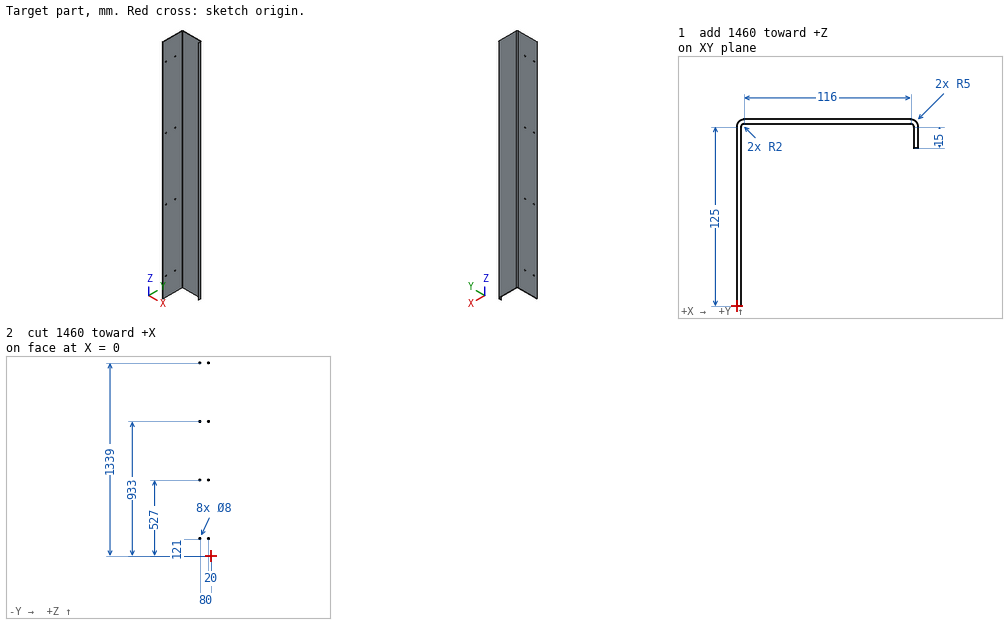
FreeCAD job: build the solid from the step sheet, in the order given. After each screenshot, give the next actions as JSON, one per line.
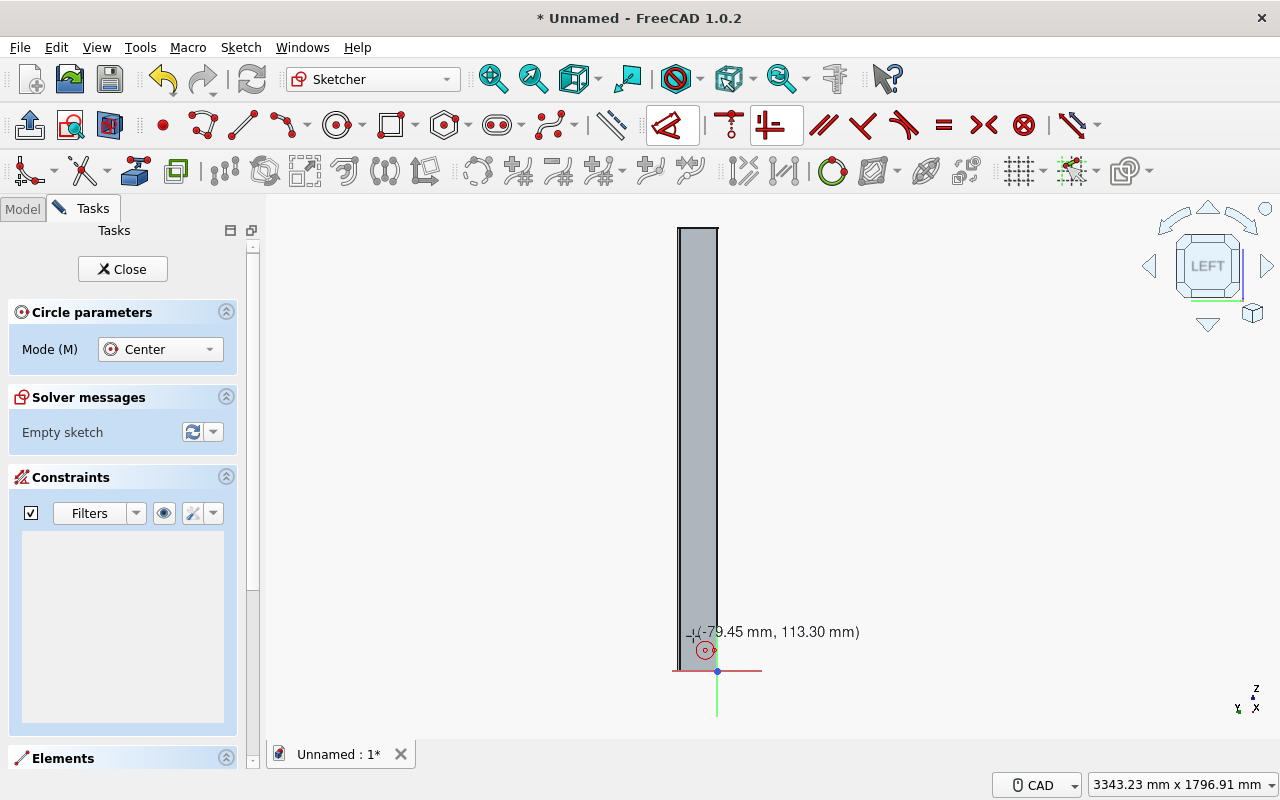
{"action": "left_click", "coordinate": [693, 634]}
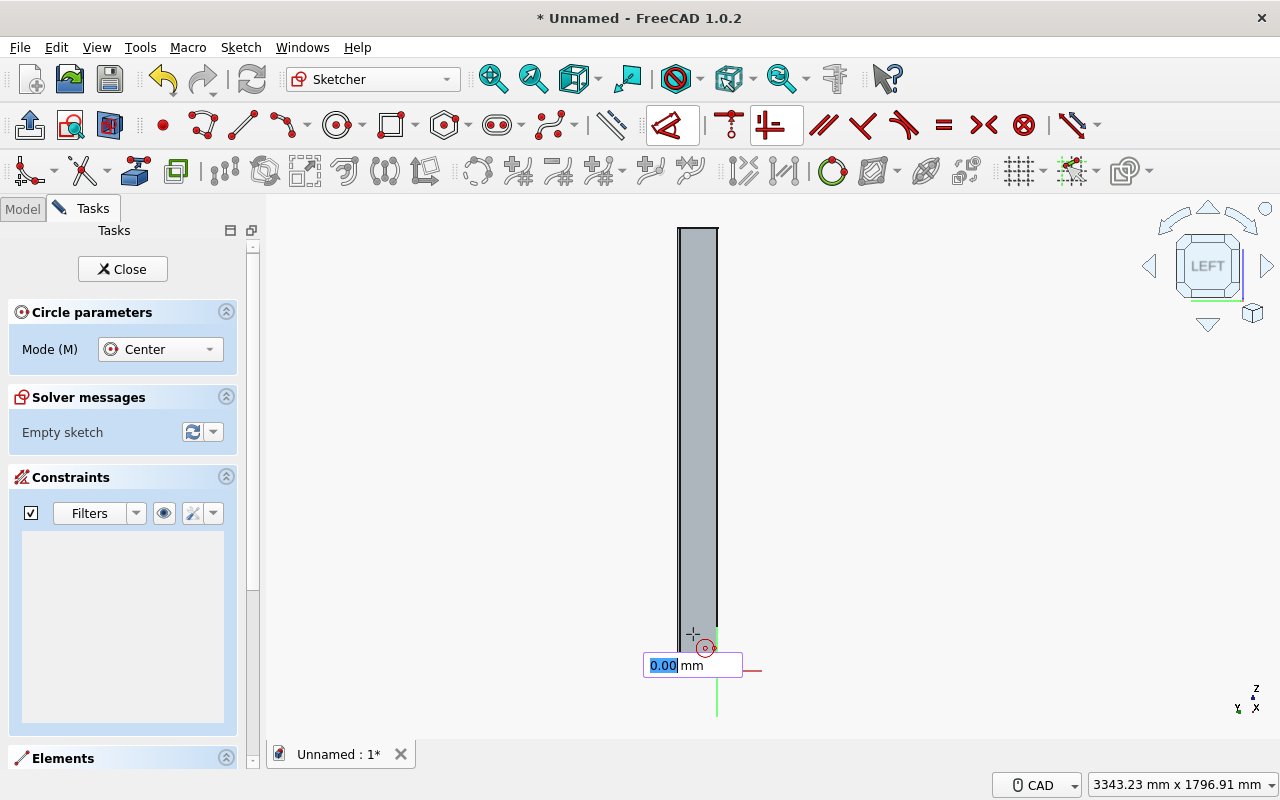
{"action": "scroll", "coordinate": [694, 634], "scroll_direction": "up", "scroll_amount": 13}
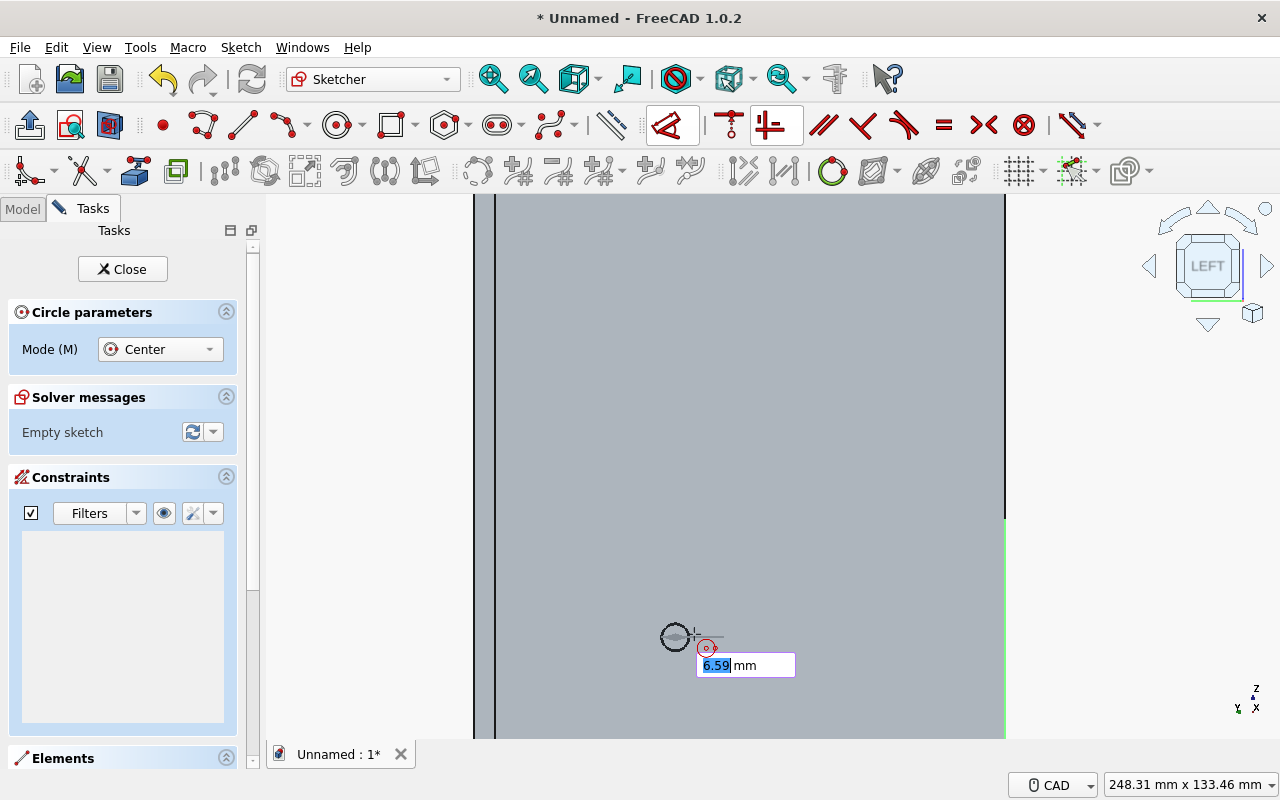
{"action": "left_click", "coordinate": [690, 619]}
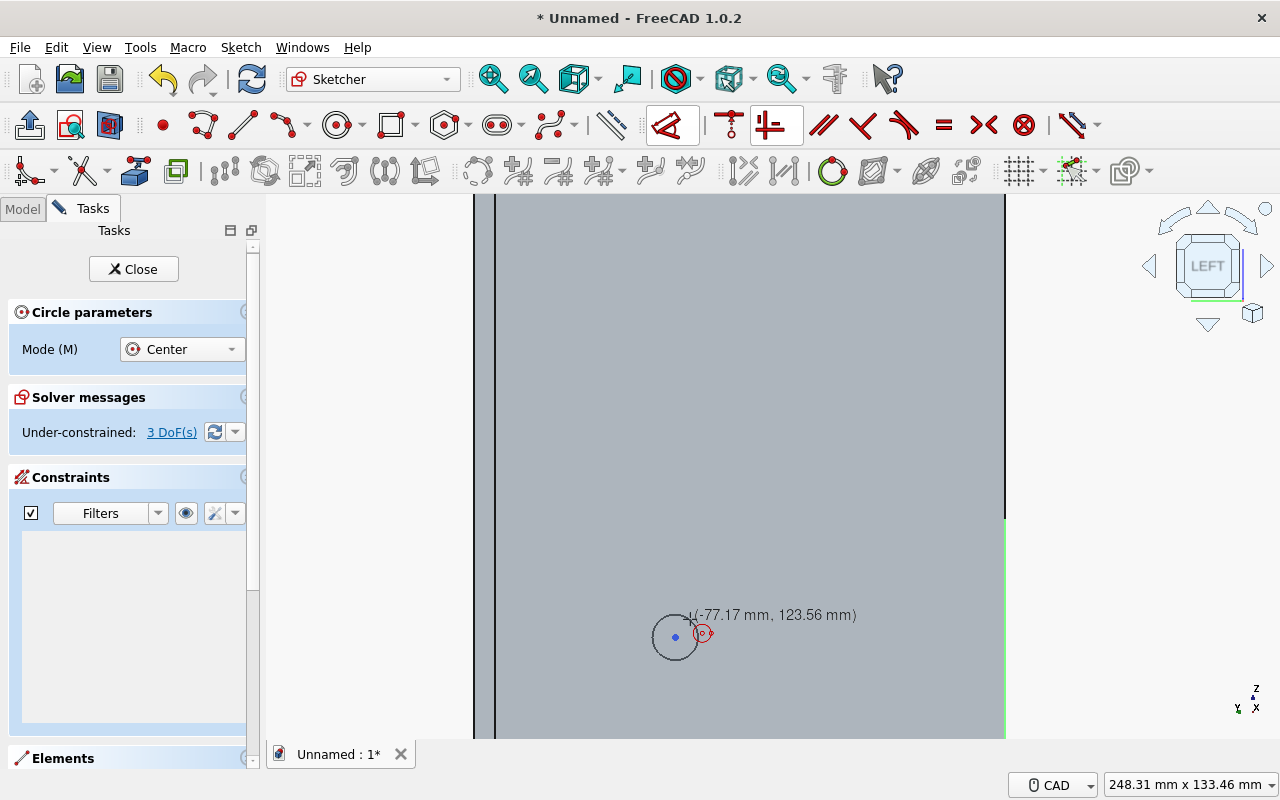
{"action": "scroll", "coordinate": [696, 601], "scroll_direction": "down", "scroll_amount": 14}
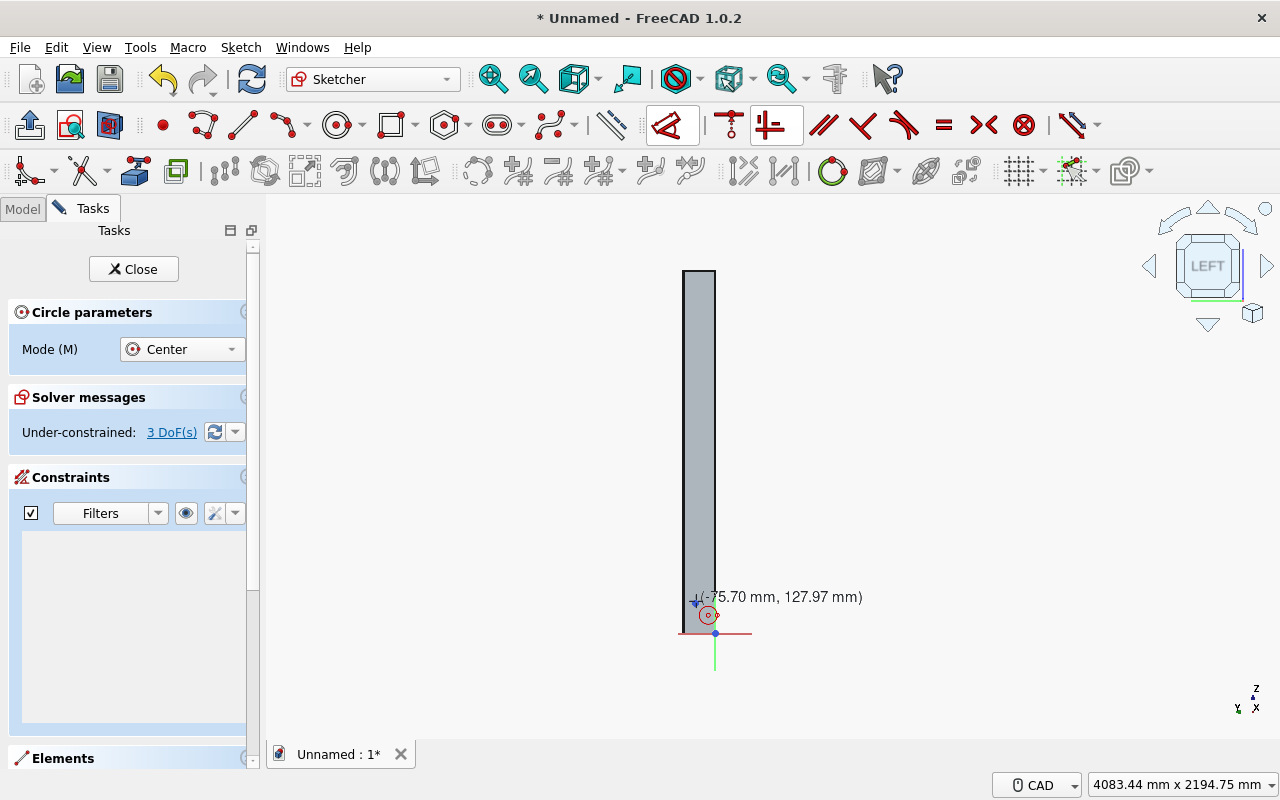
{"action": "scroll", "coordinate": [695, 301], "scroll_direction": "up", "scroll_amount": 16}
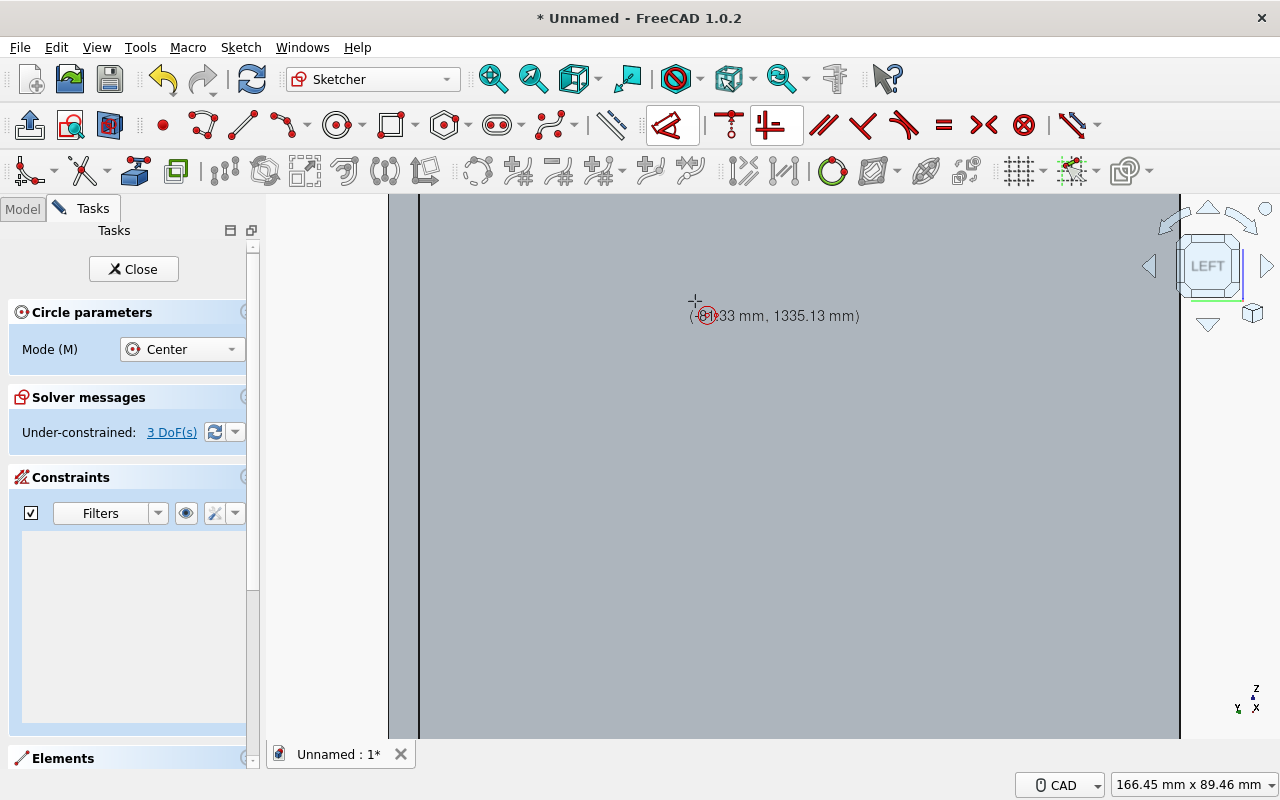
{"action": "scroll", "coordinate": [693, 262], "scroll_direction": "down", "scroll_amount": 15}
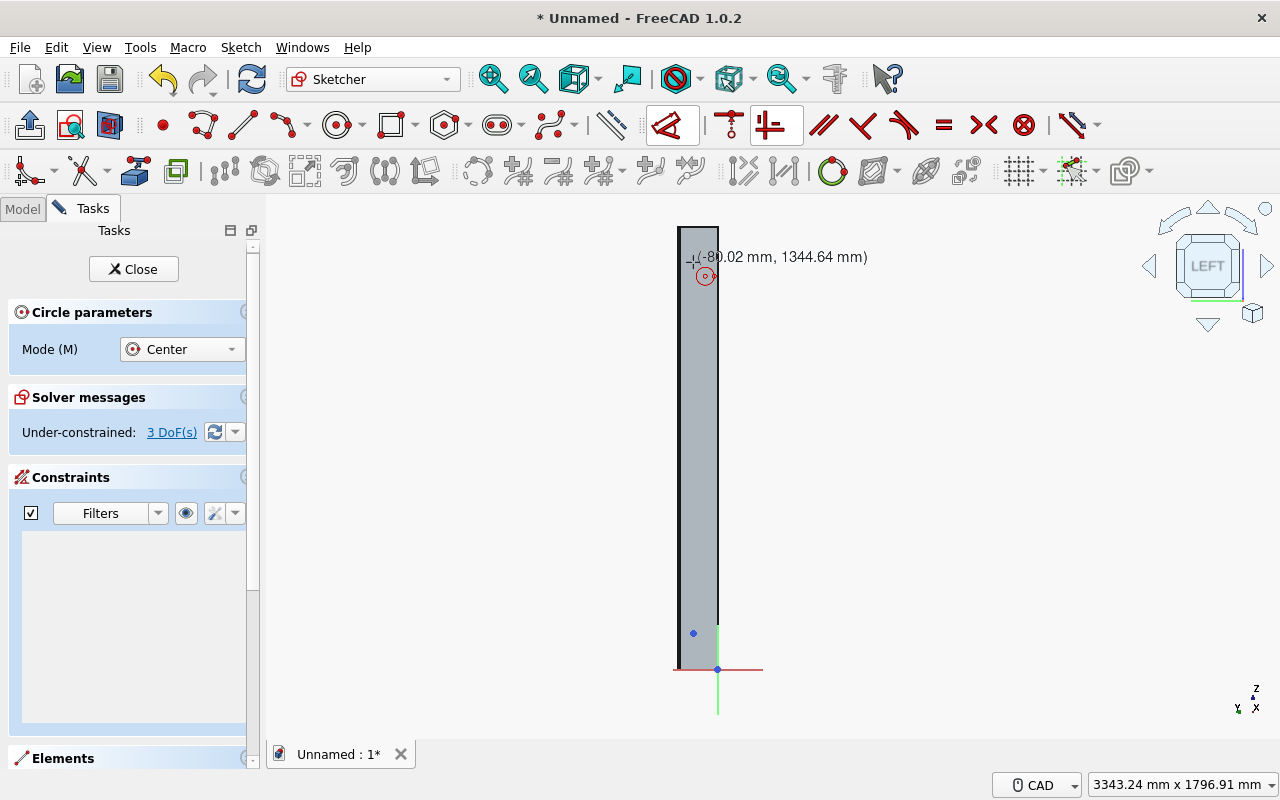
{"action": "left_click", "coordinate": [693, 264]}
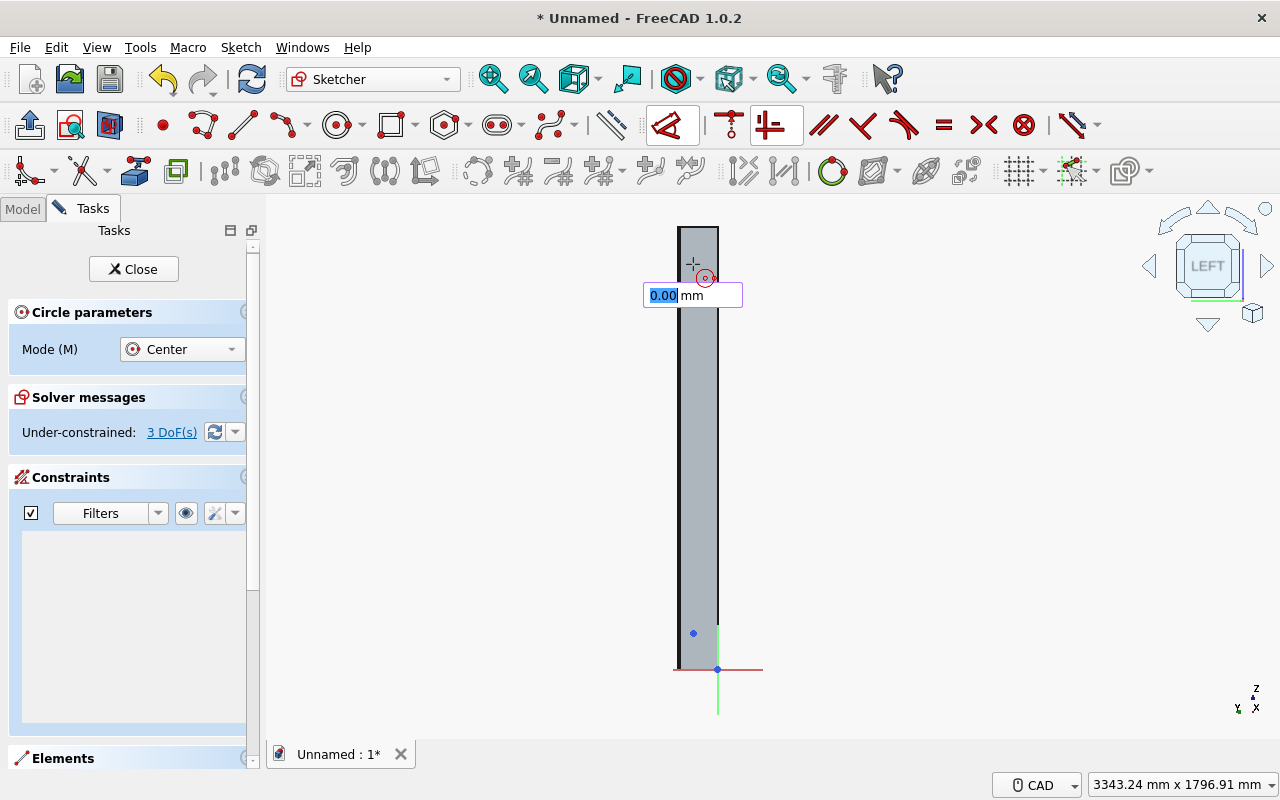
{"action": "scroll", "coordinate": [694, 263], "scroll_direction": "up", "scroll_amount": 13}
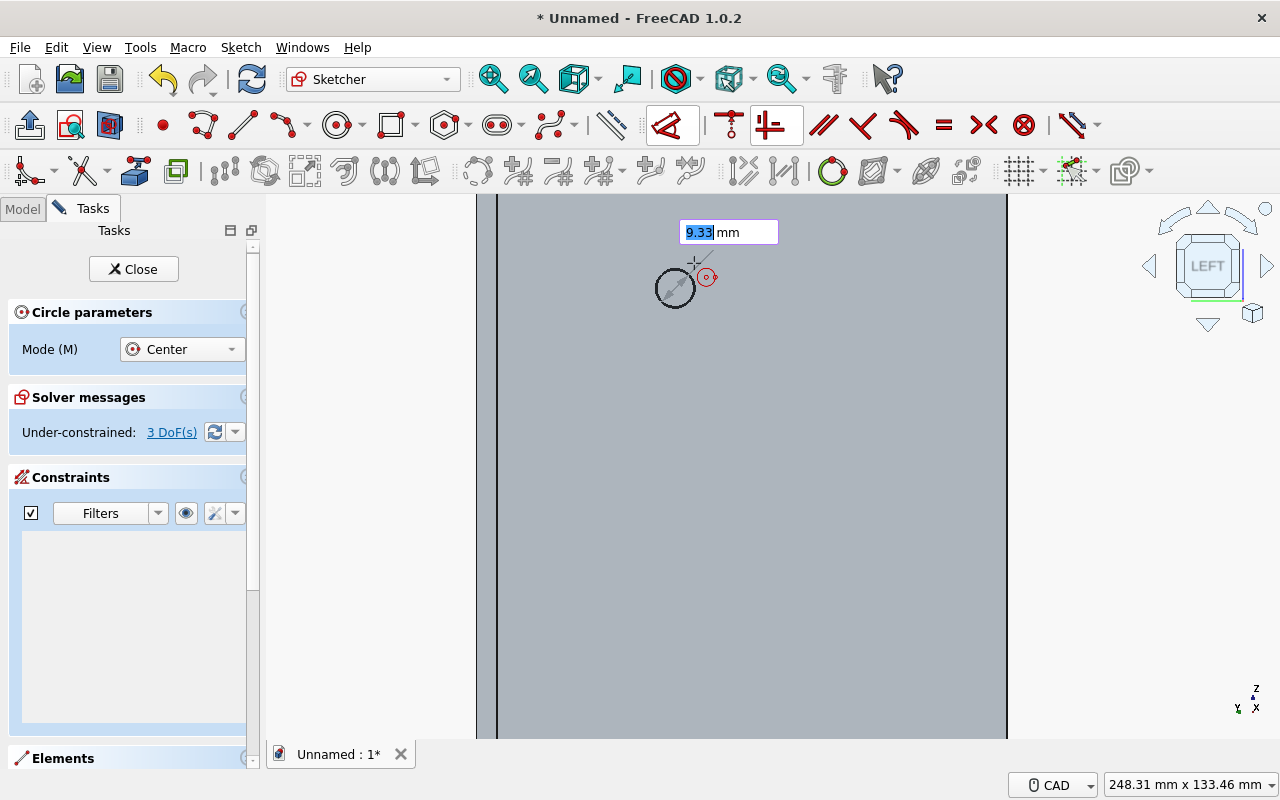
{"action": "left_click", "coordinate": [692, 262]}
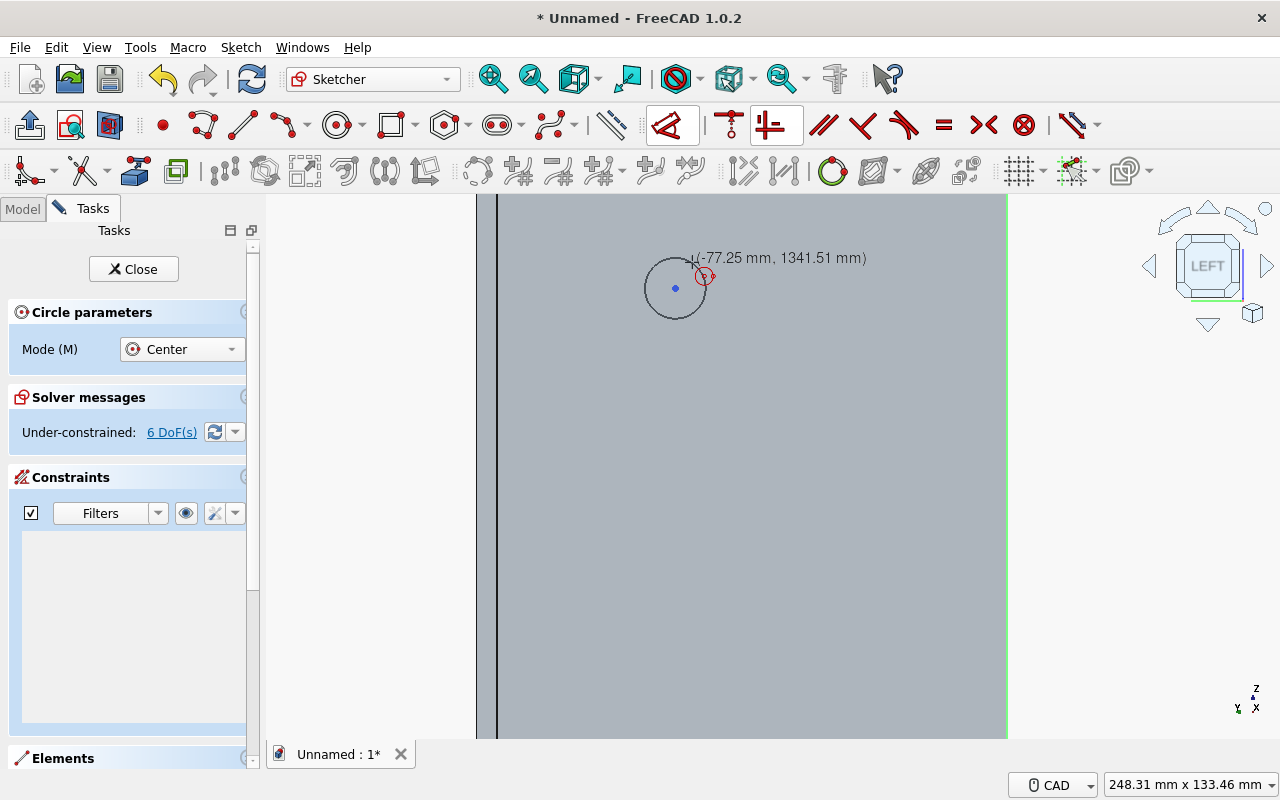
{"action": "scroll", "coordinate": [696, 303], "scroll_direction": "down", "scroll_amount": 14}